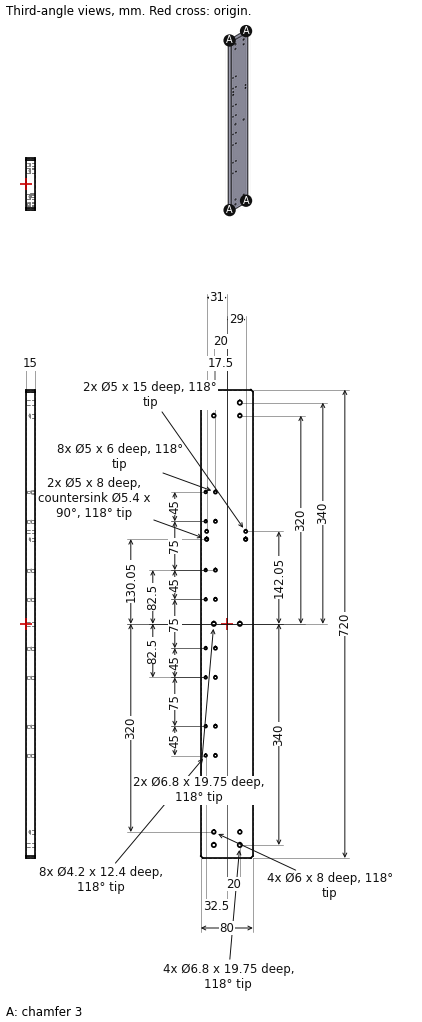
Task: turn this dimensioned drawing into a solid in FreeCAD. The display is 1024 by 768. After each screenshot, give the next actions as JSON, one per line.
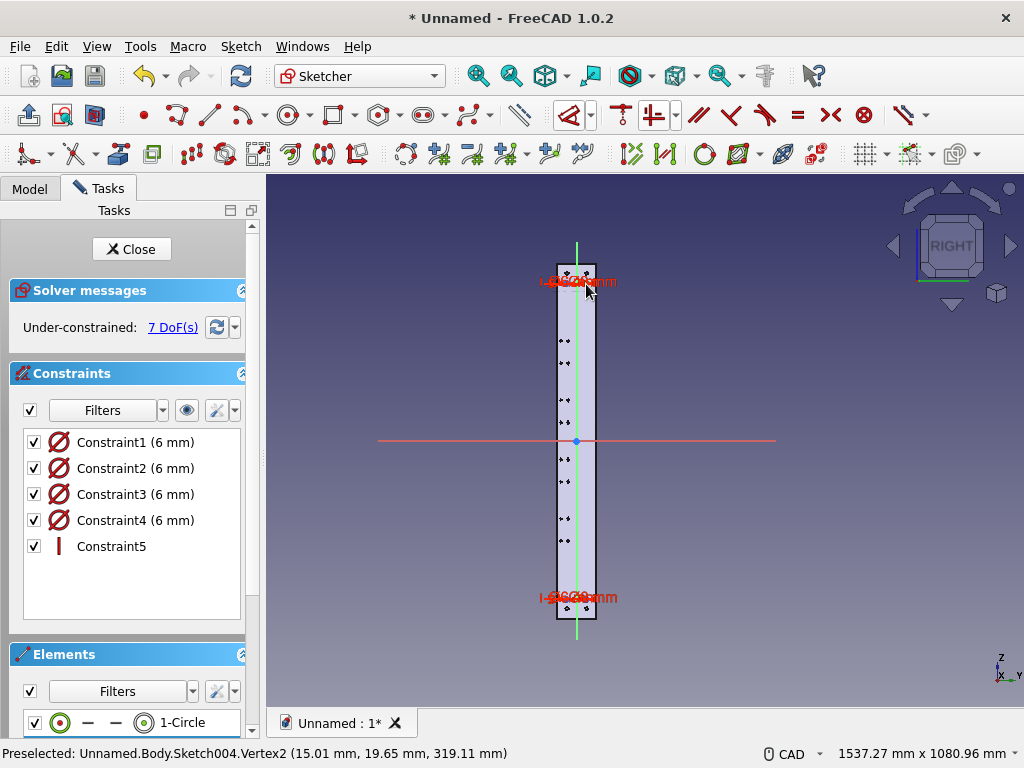
{"action": "left_click", "coordinate": [567, 284]}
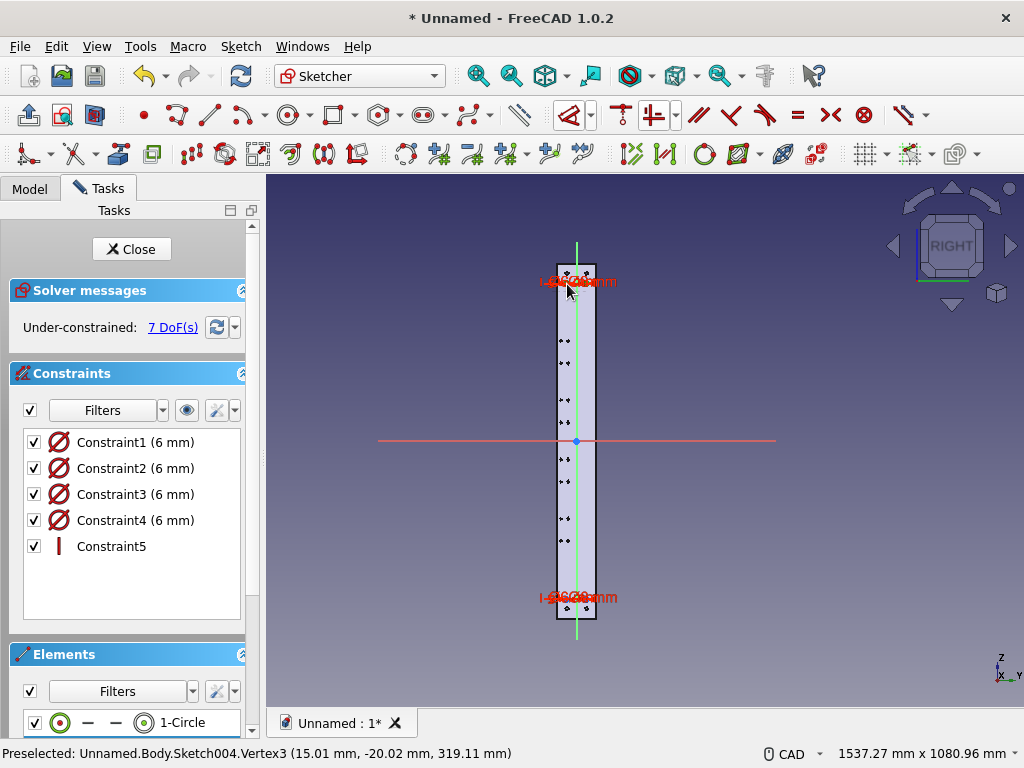
{"action": "key", "text": "h"}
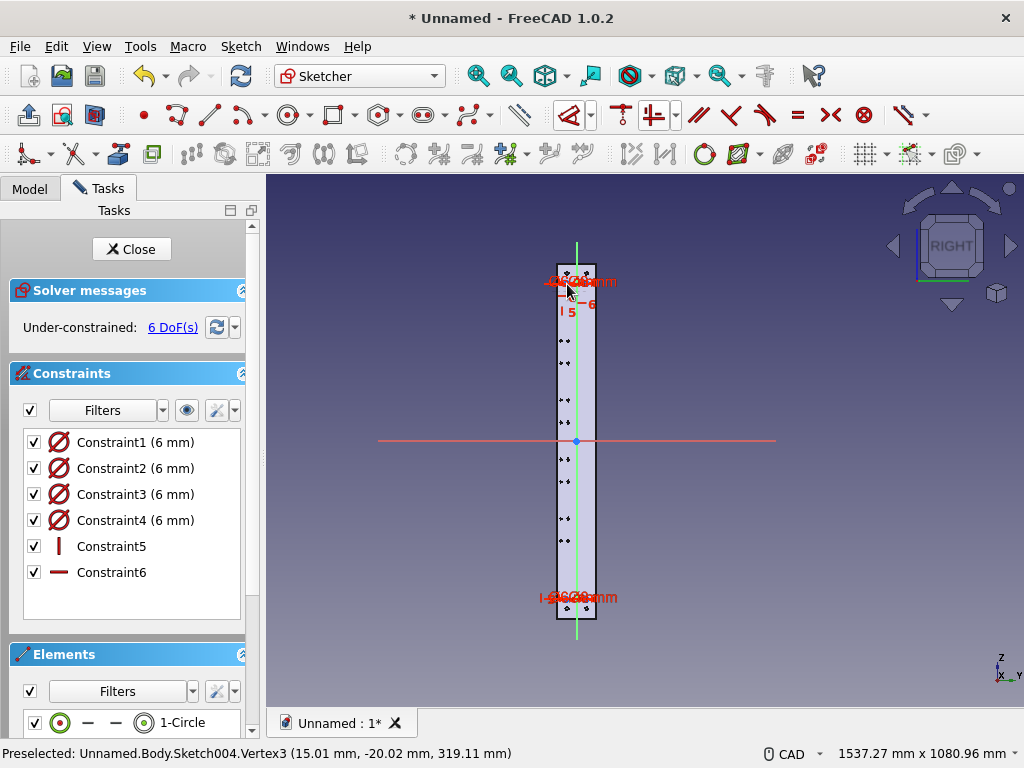
{"action": "left_click", "coordinate": [586, 284]}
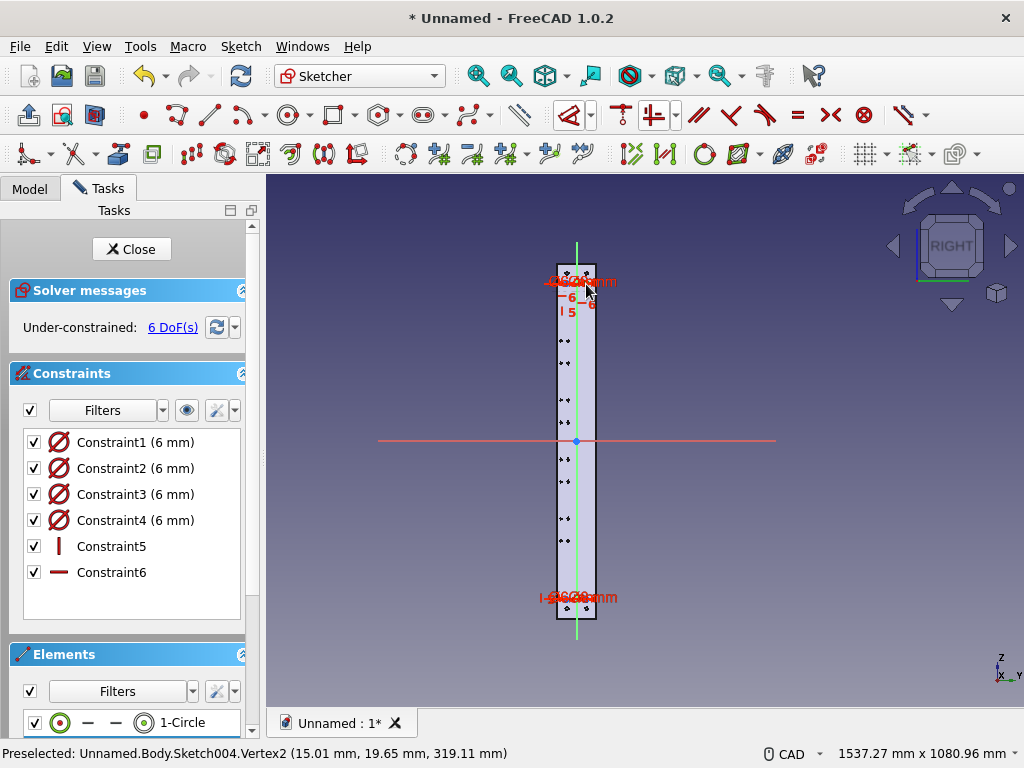
{"action": "left_click", "coordinate": [587, 599]}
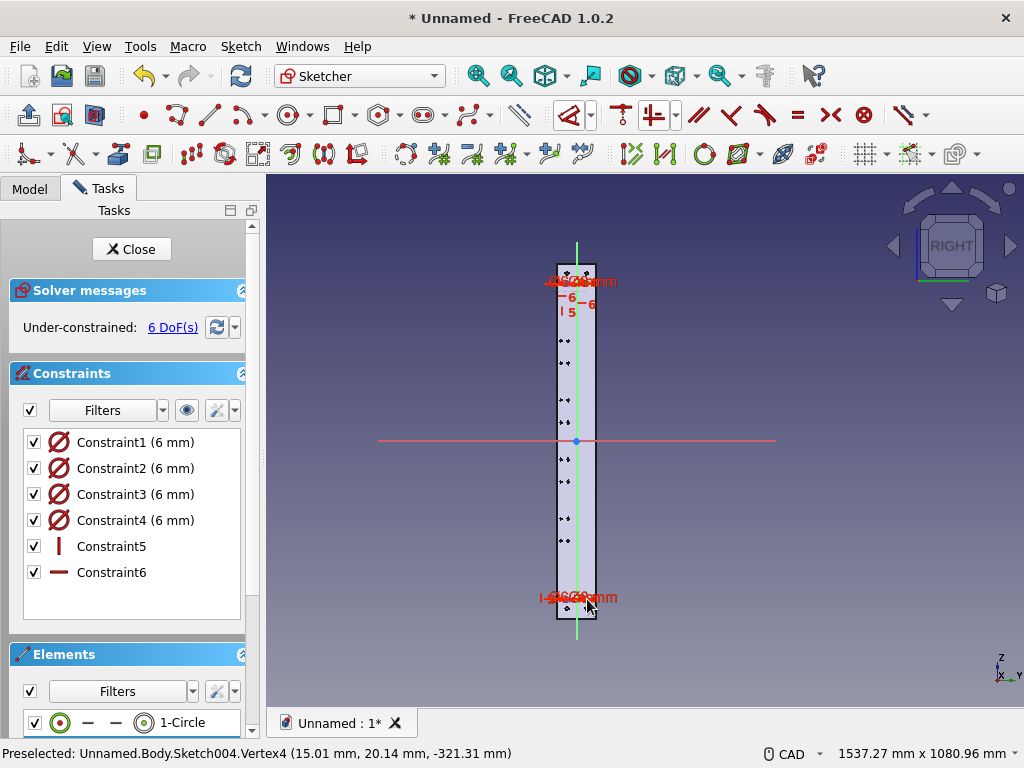
{"action": "key", "text": "v"}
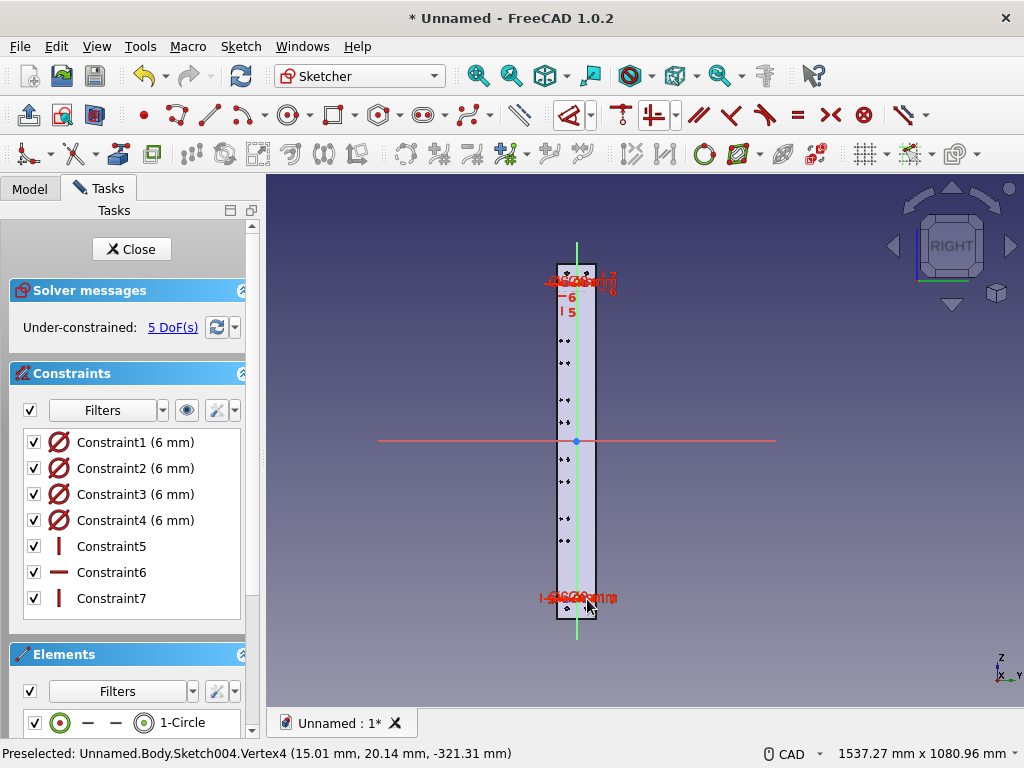
{"action": "left_click", "coordinate": [567, 599]}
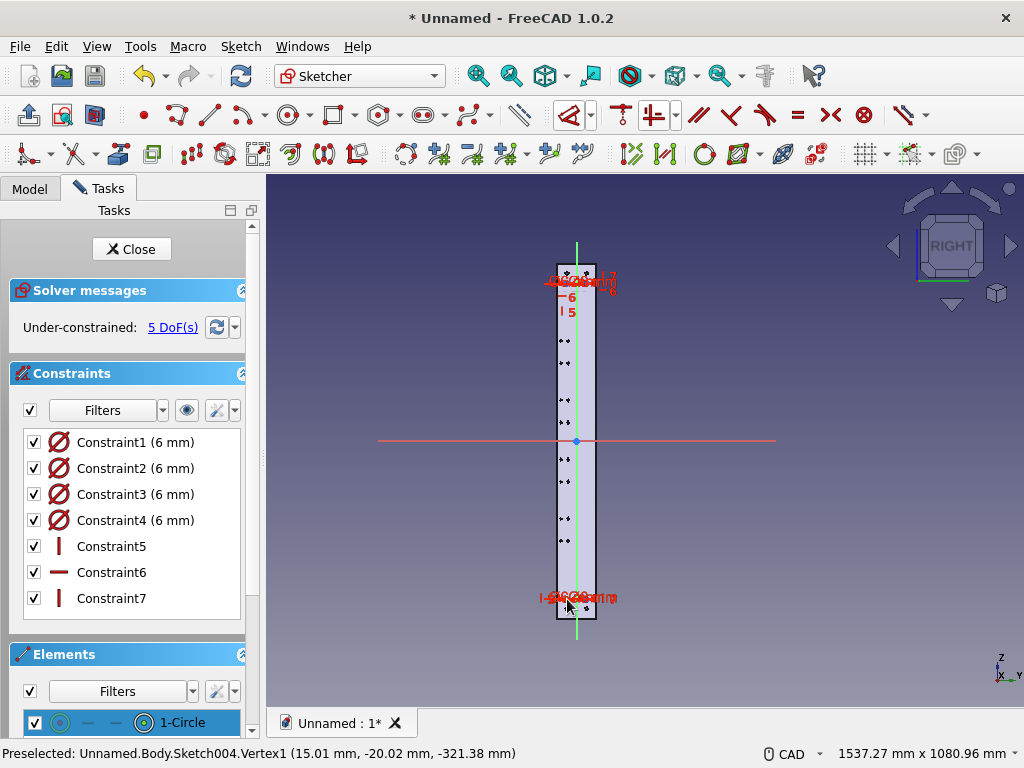
{"action": "left_click", "coordinate": [586, 599]}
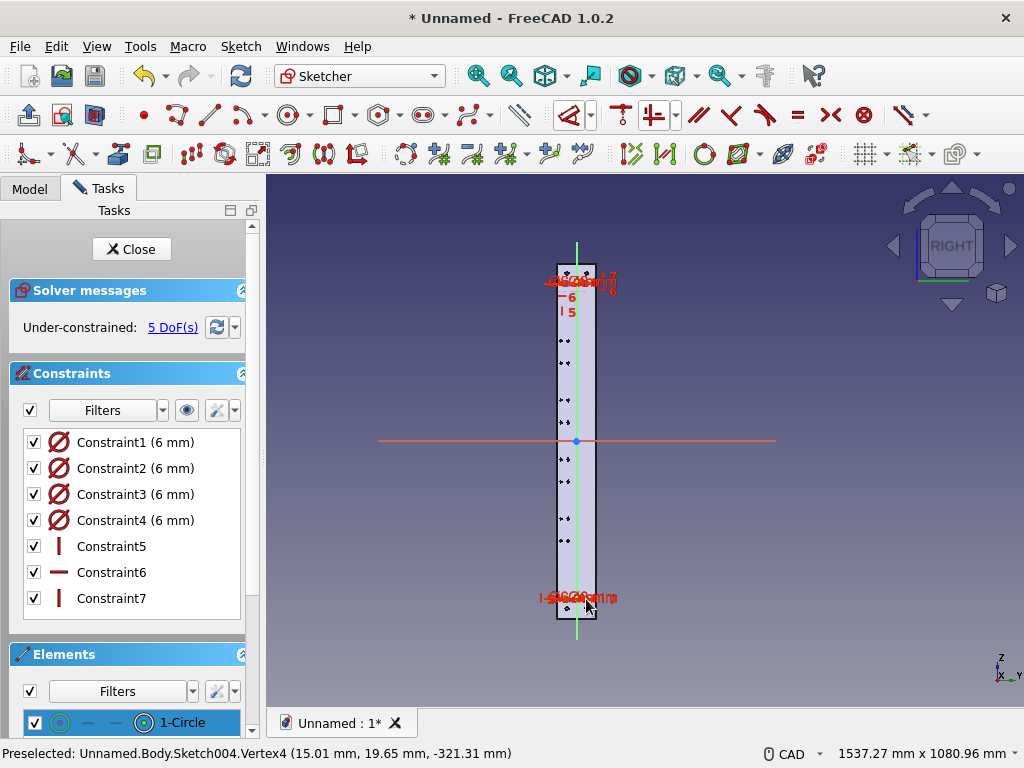
{"action": "left_click", "coordinate": [676, 116]}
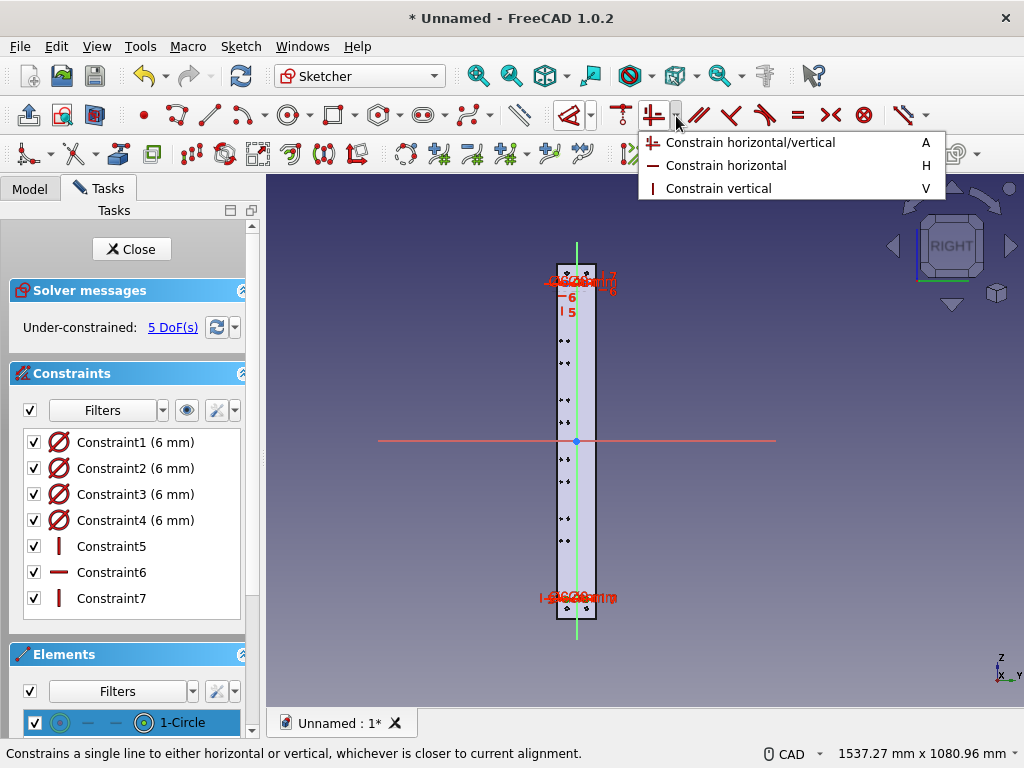
{"action": "left_click", "coordinate": [792, 166]}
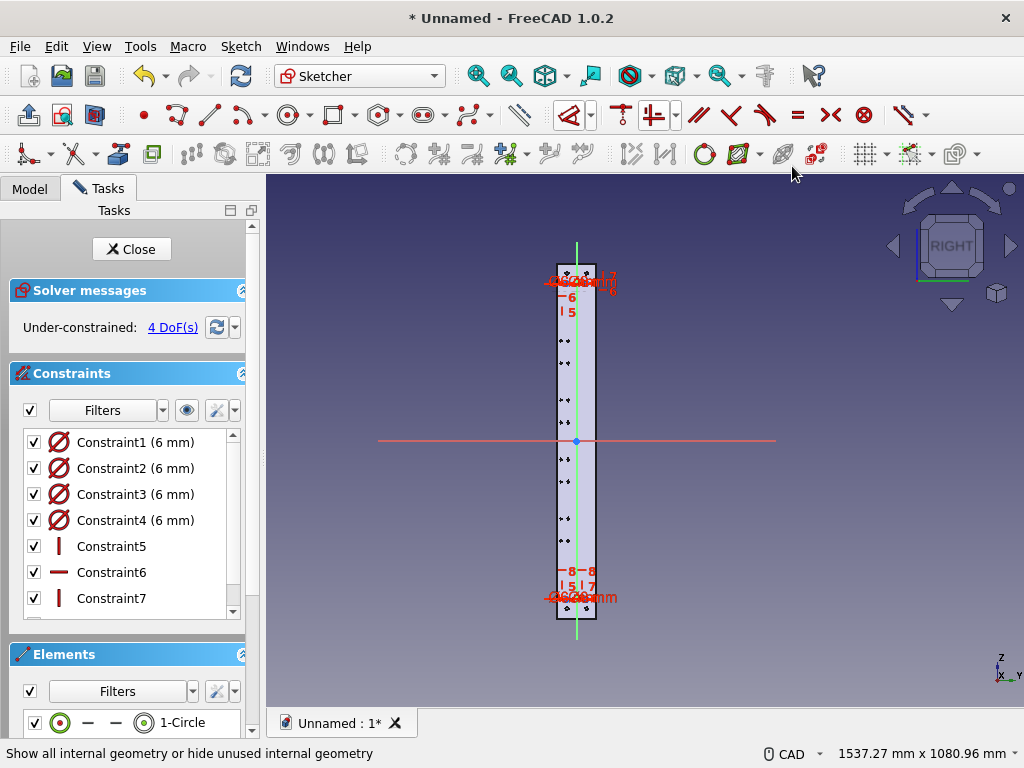
{"action": "scroll", "coordinate": [567, 599], "scroll_direction": "up", "scroll_amount": 7}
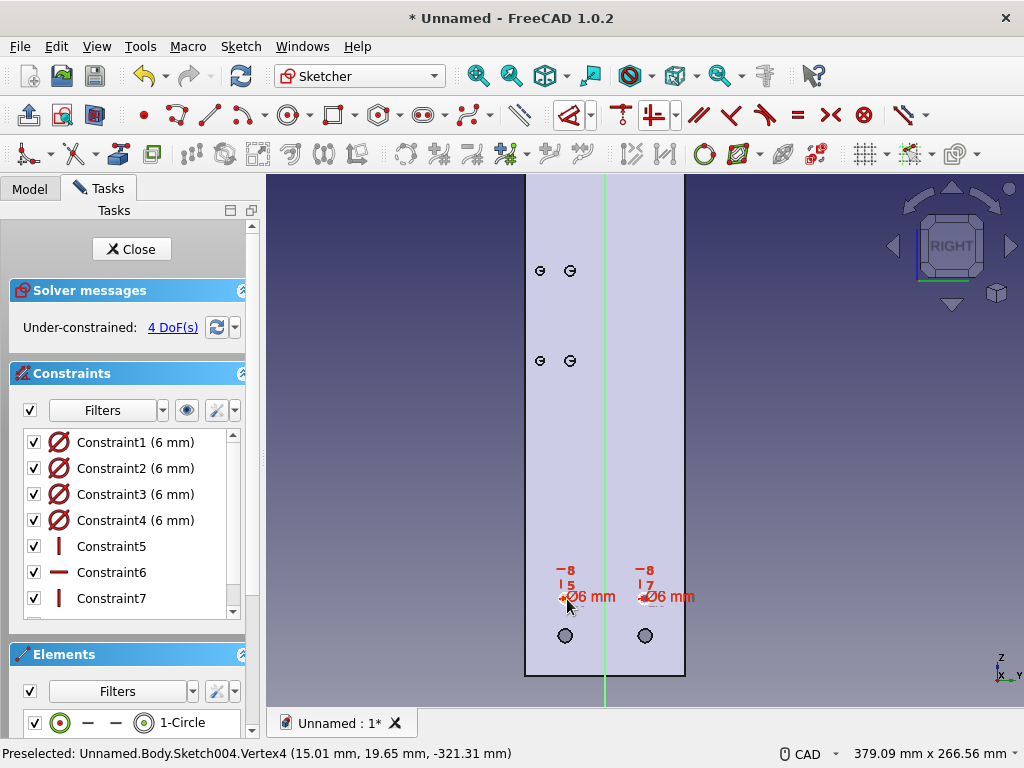
{"action": "left_click", "coordinate": [565, 599]}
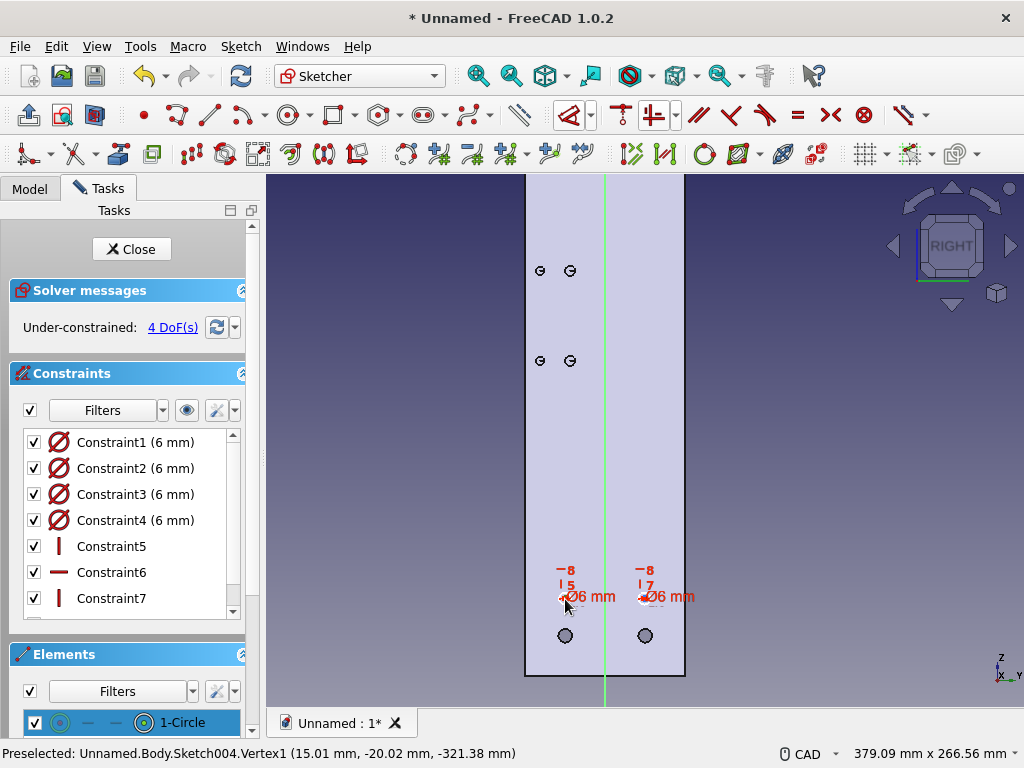
{"action": "key", "text": "l"}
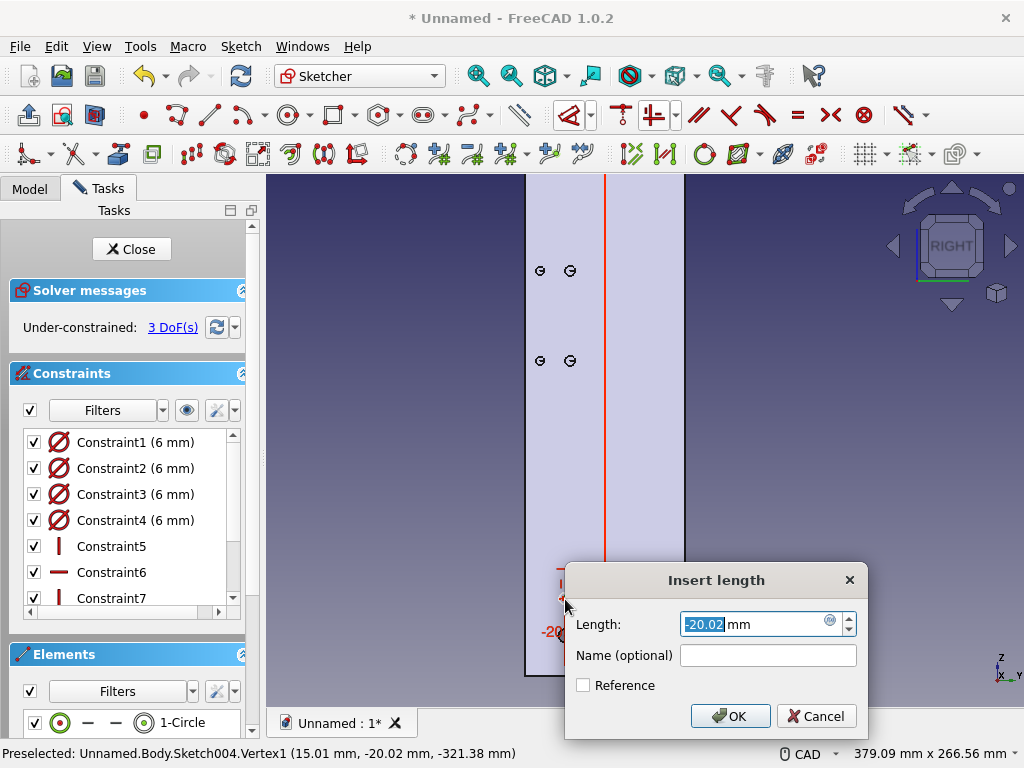
{"action": "type", "text": "-20"}
{"action": "key", "text": "Return"}